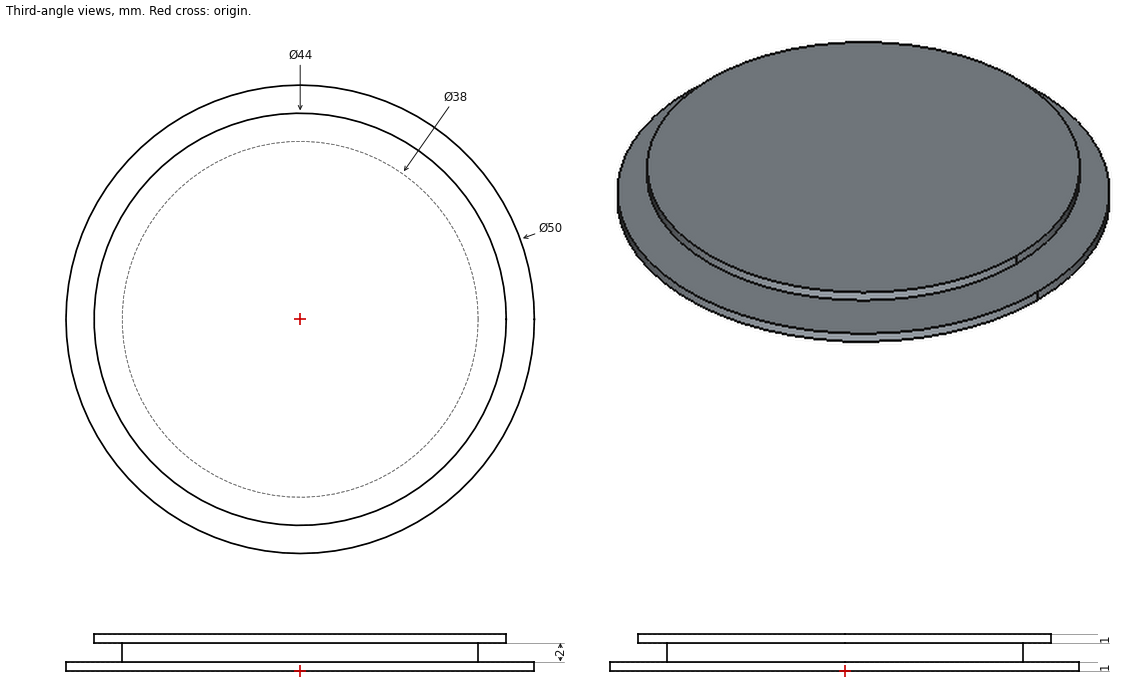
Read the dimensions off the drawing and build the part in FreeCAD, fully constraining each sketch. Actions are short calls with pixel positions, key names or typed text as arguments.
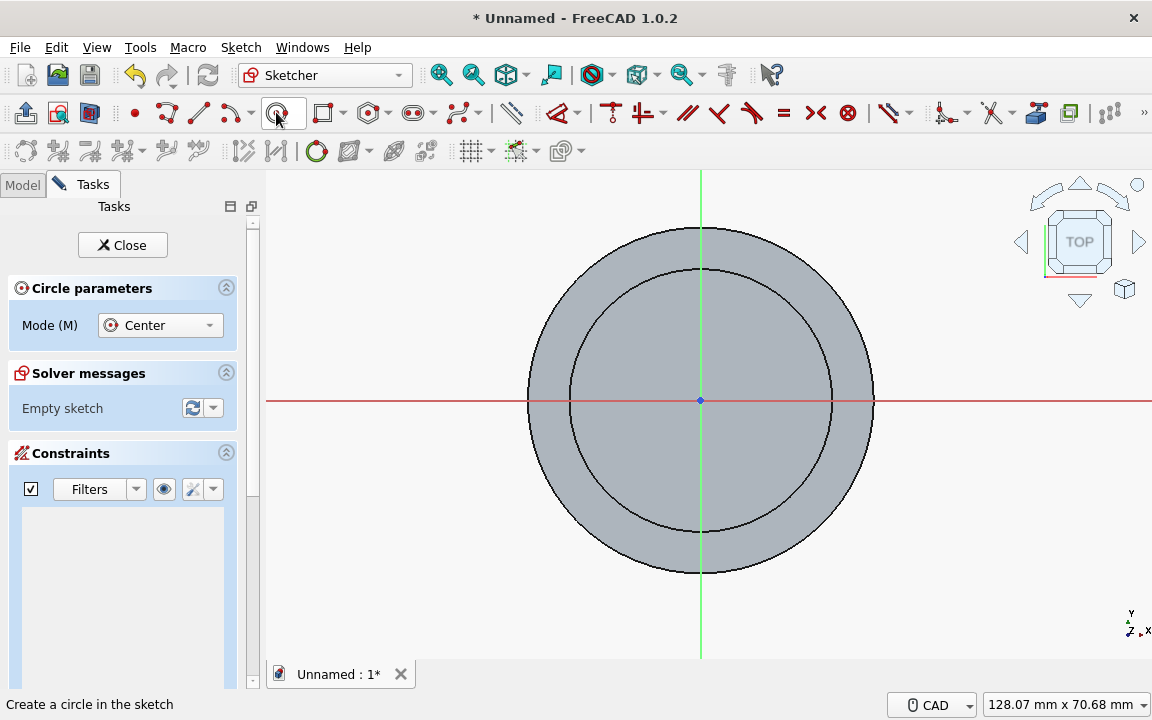
click(701, 401)
move(808, 293)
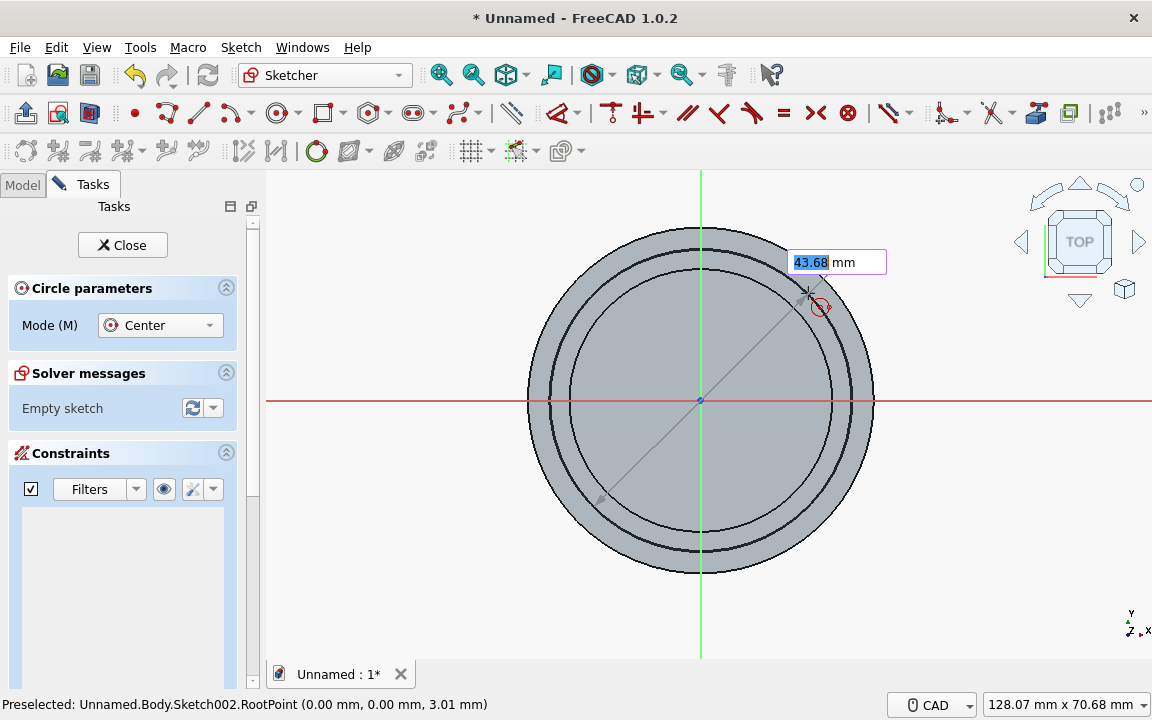
text(44)
key(Return)
key(Escape)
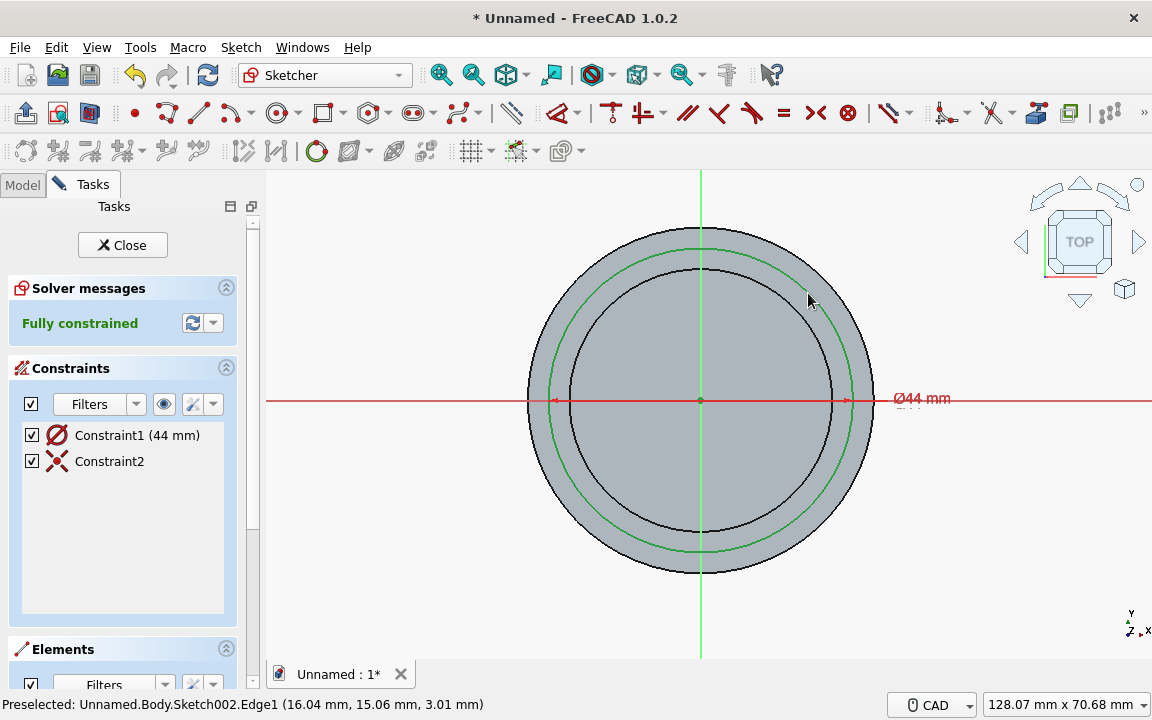
click(123, 245)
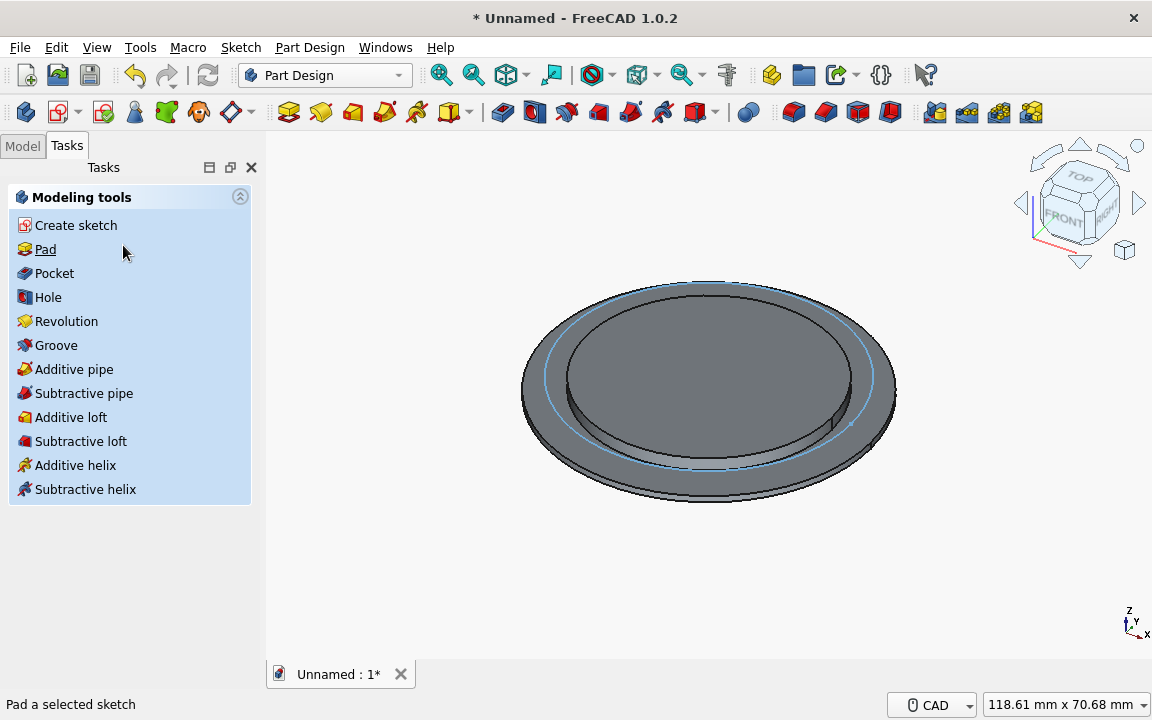
click(290, 112)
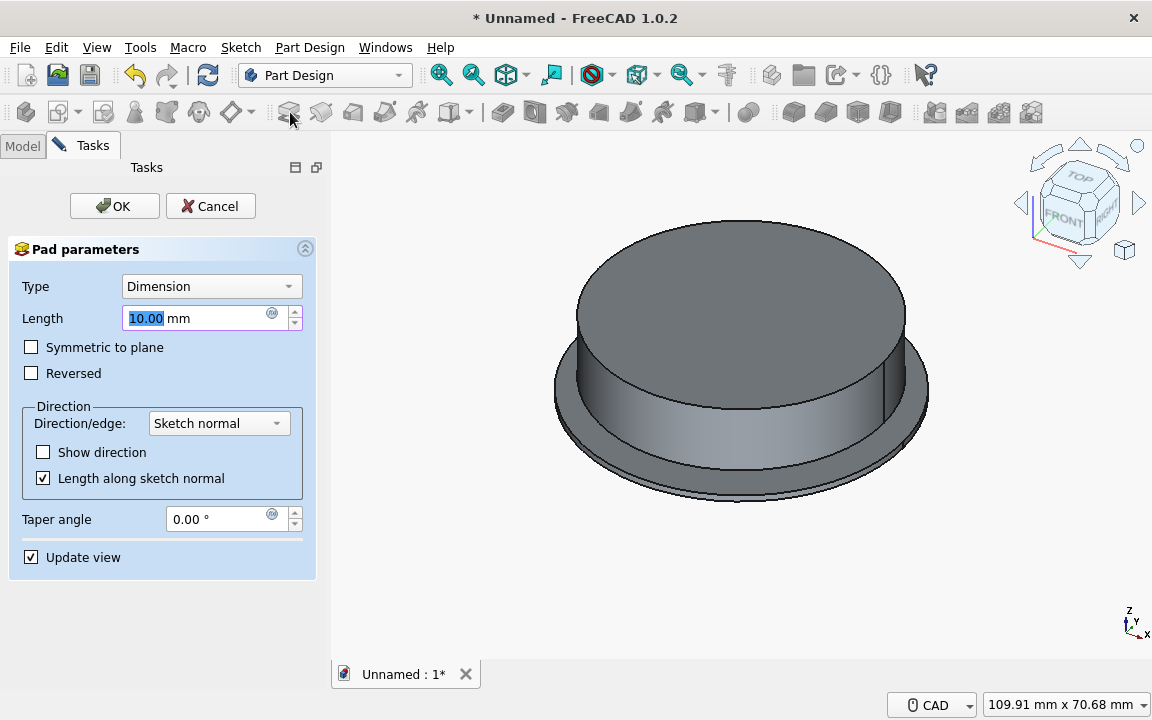
text(1)
key(Tab)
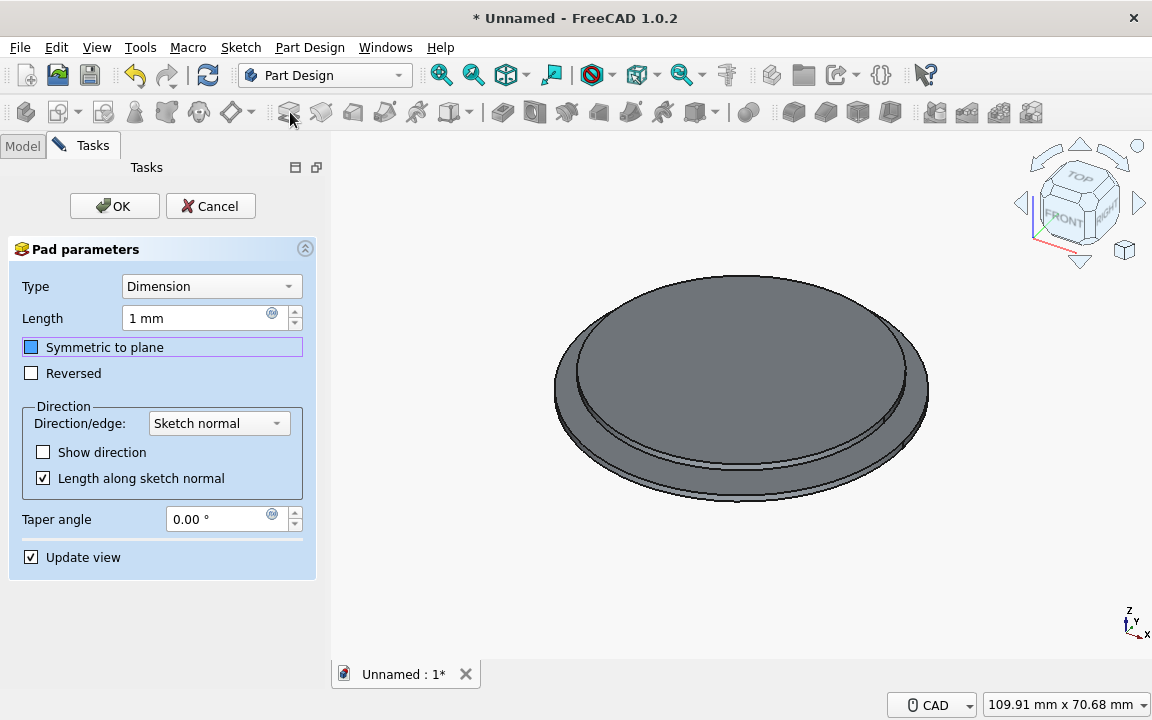
click(115, 206)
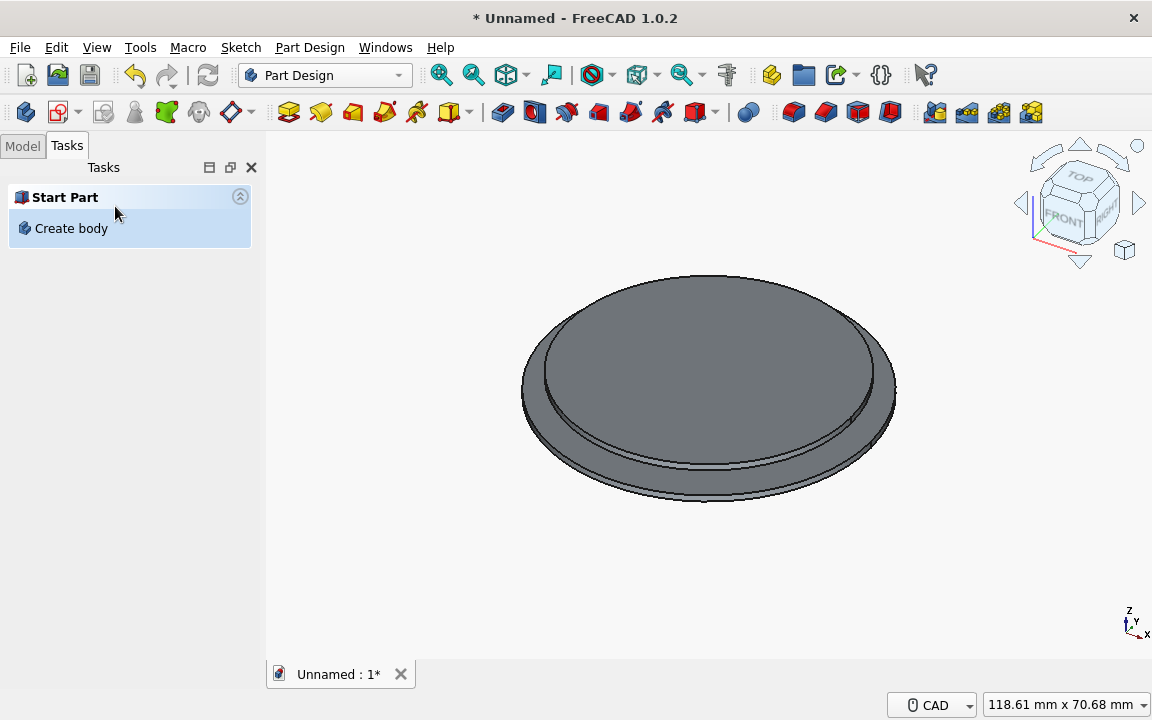
key(0)